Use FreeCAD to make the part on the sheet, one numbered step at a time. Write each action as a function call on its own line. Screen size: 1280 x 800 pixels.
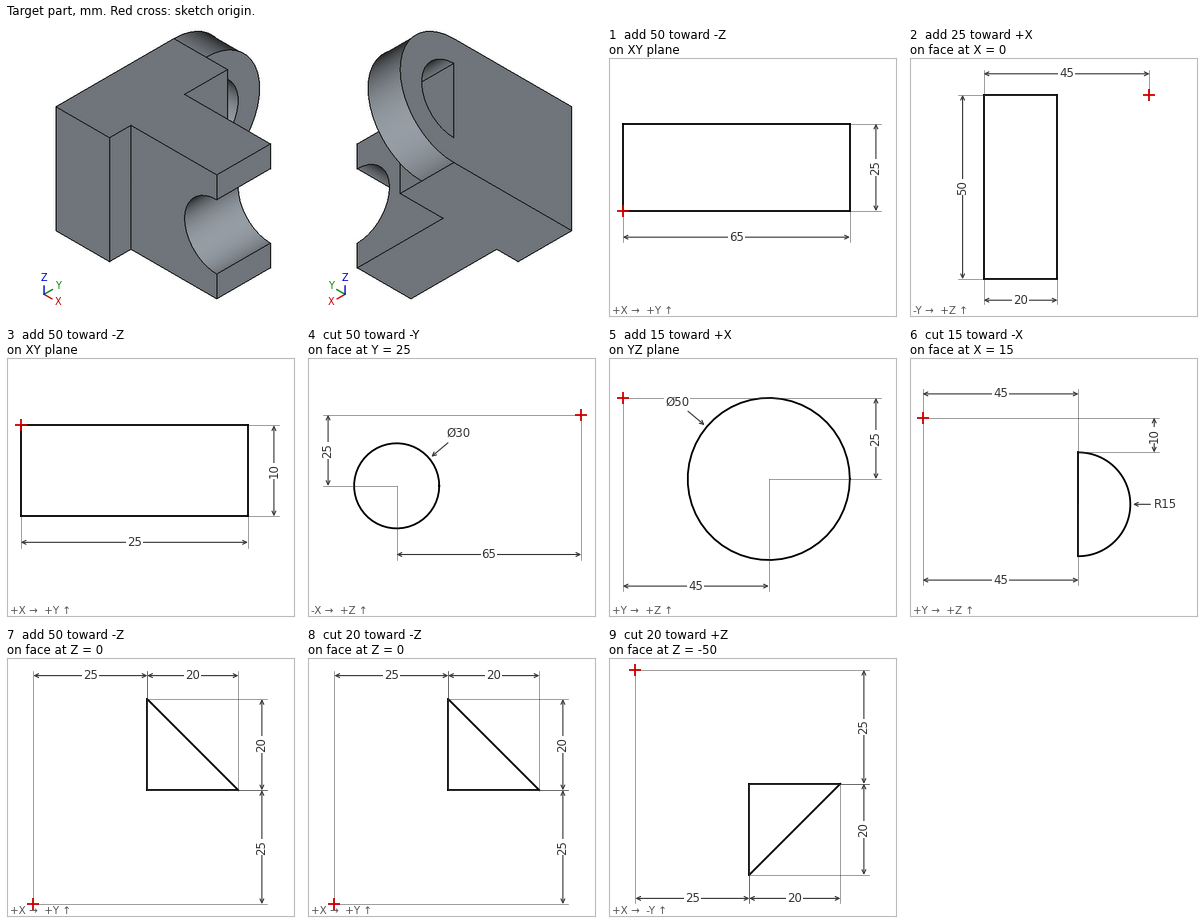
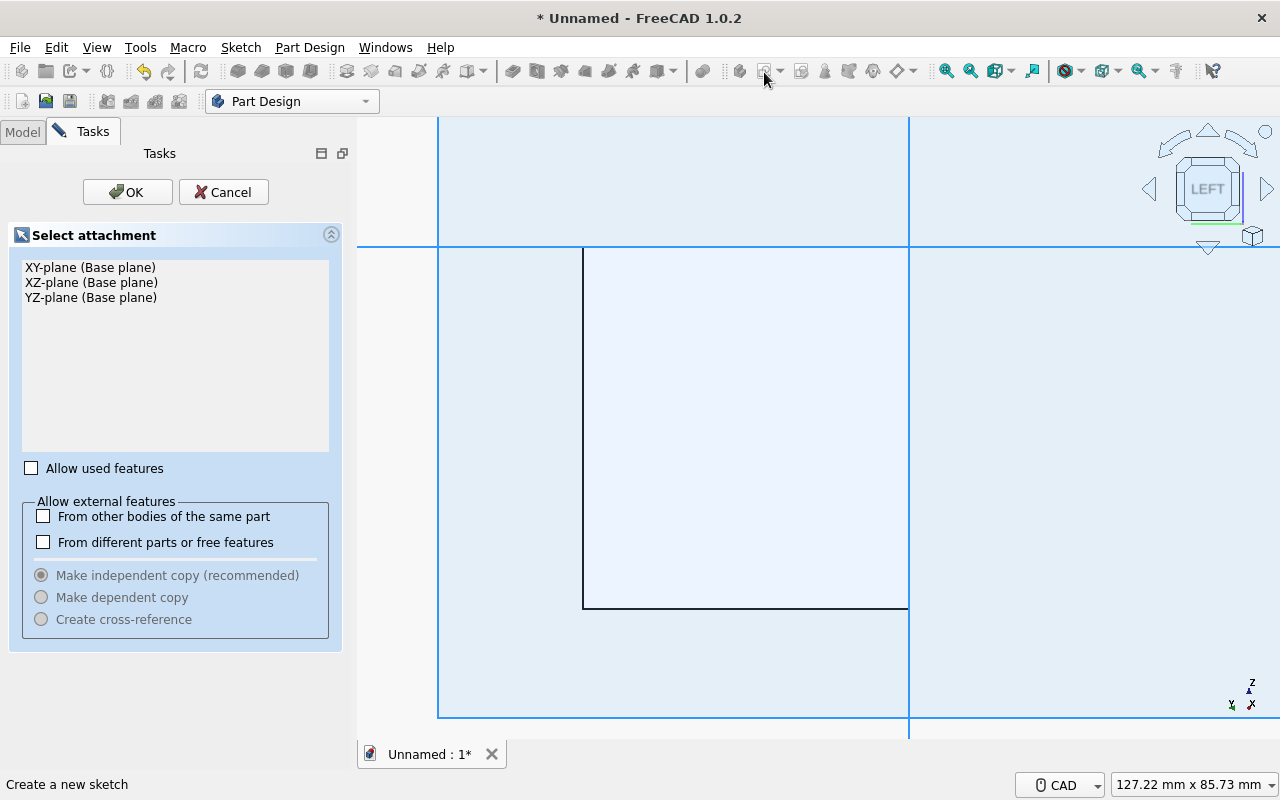
click(82, 268)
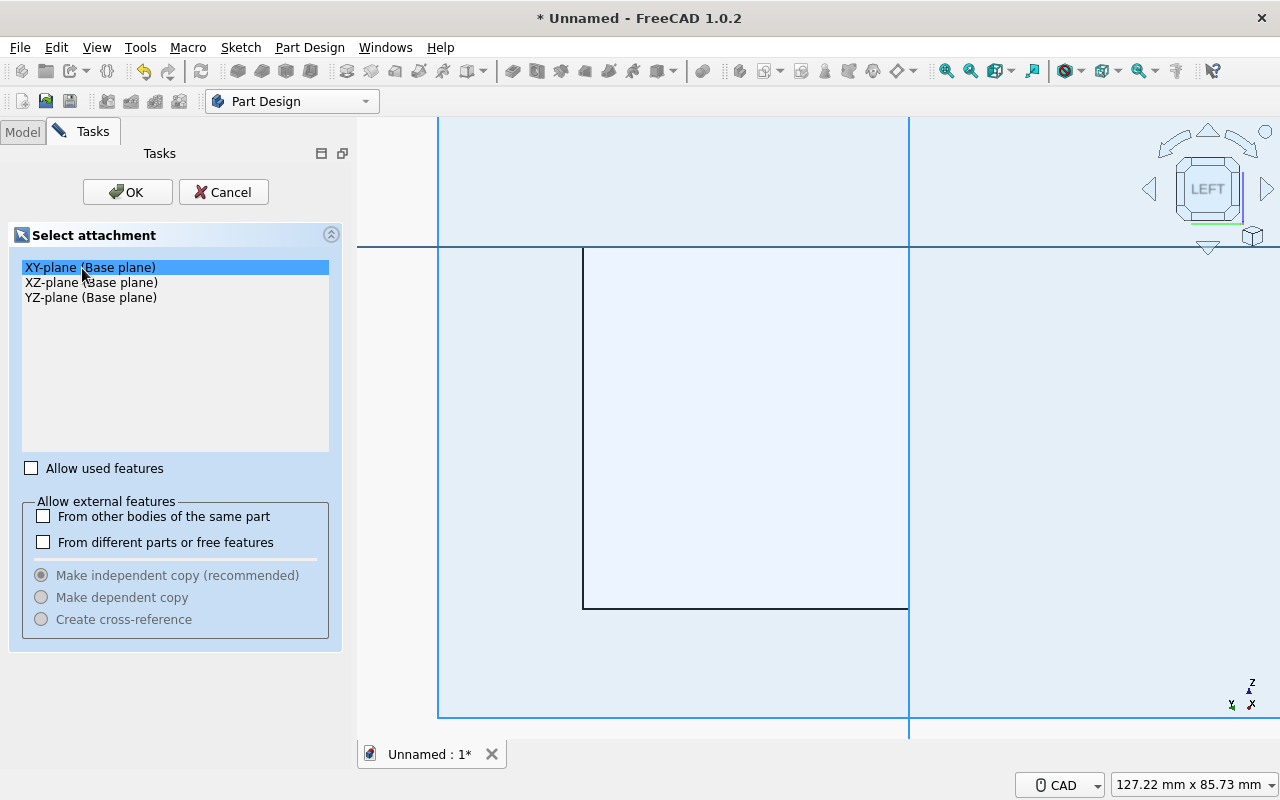
click(128, 192)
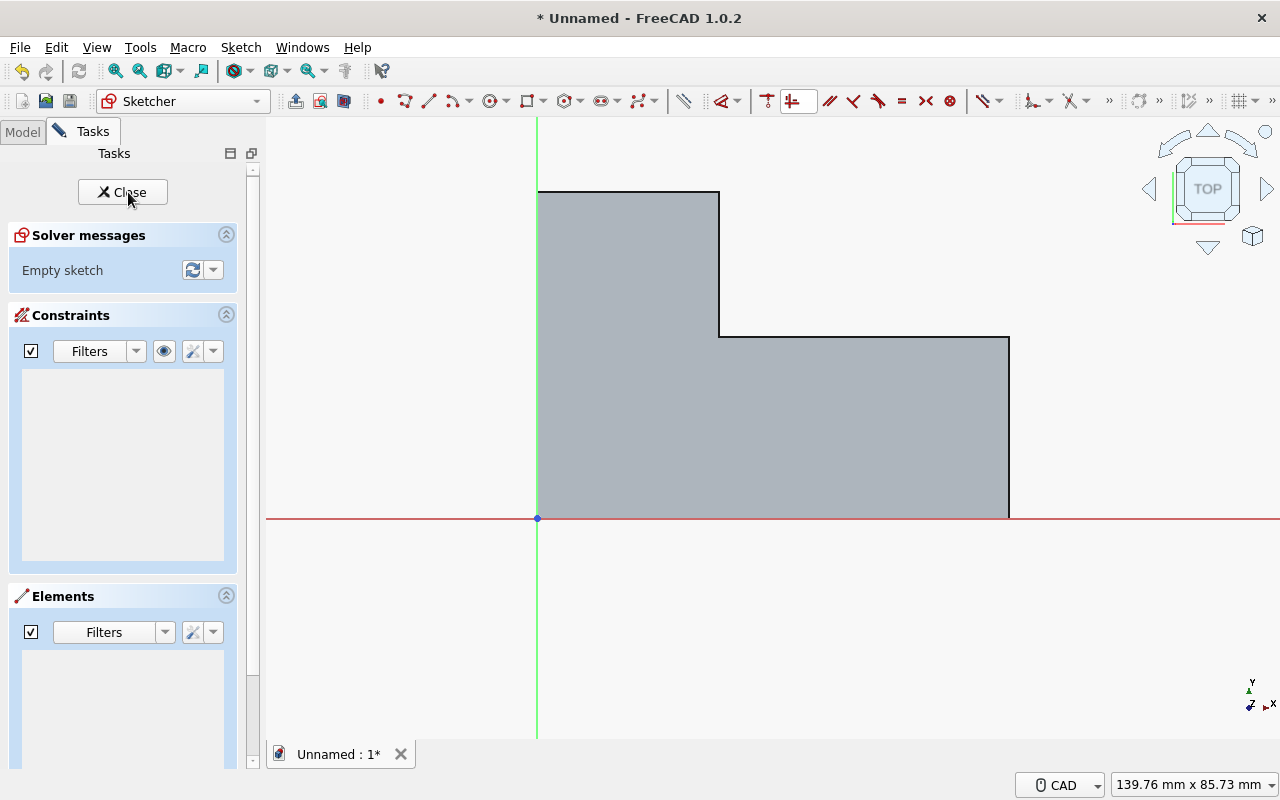
scroll(595, 610, up, 6)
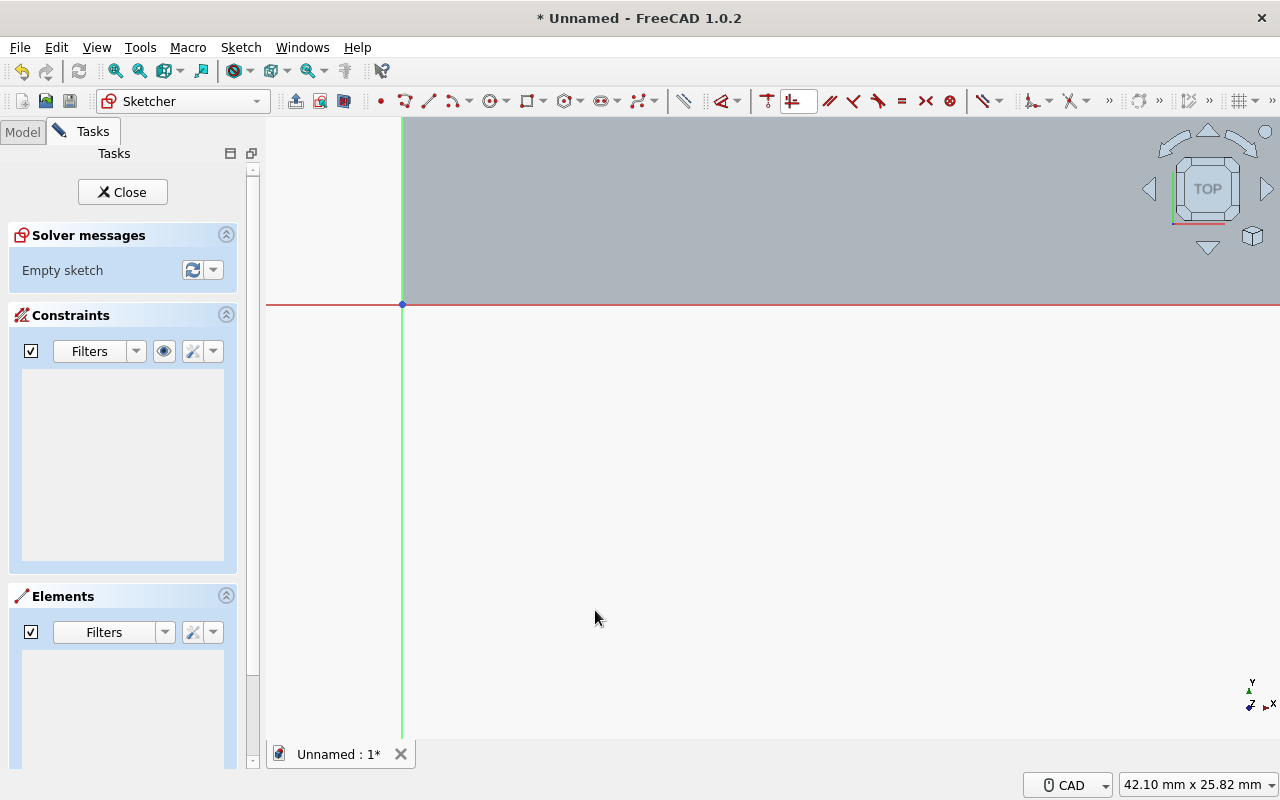
click(528, 102)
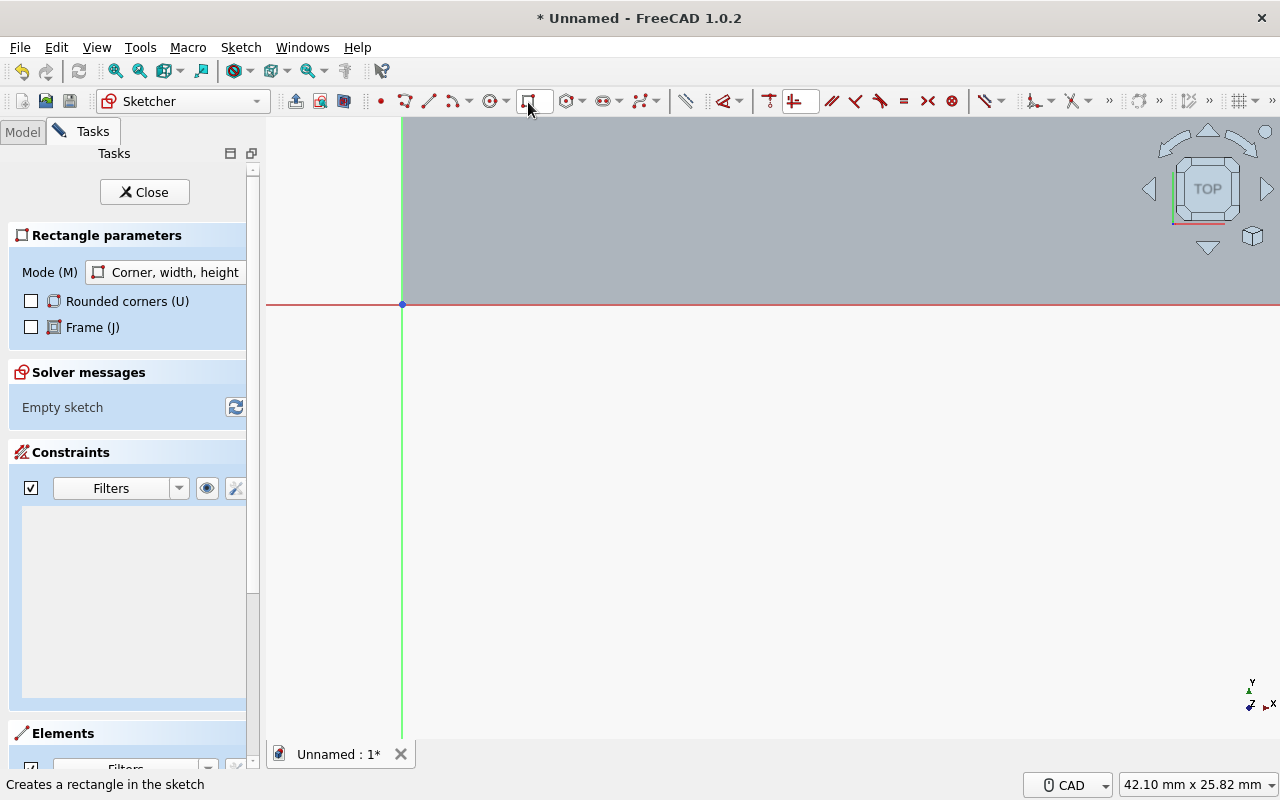
click(402, 305)
move(1005, 546)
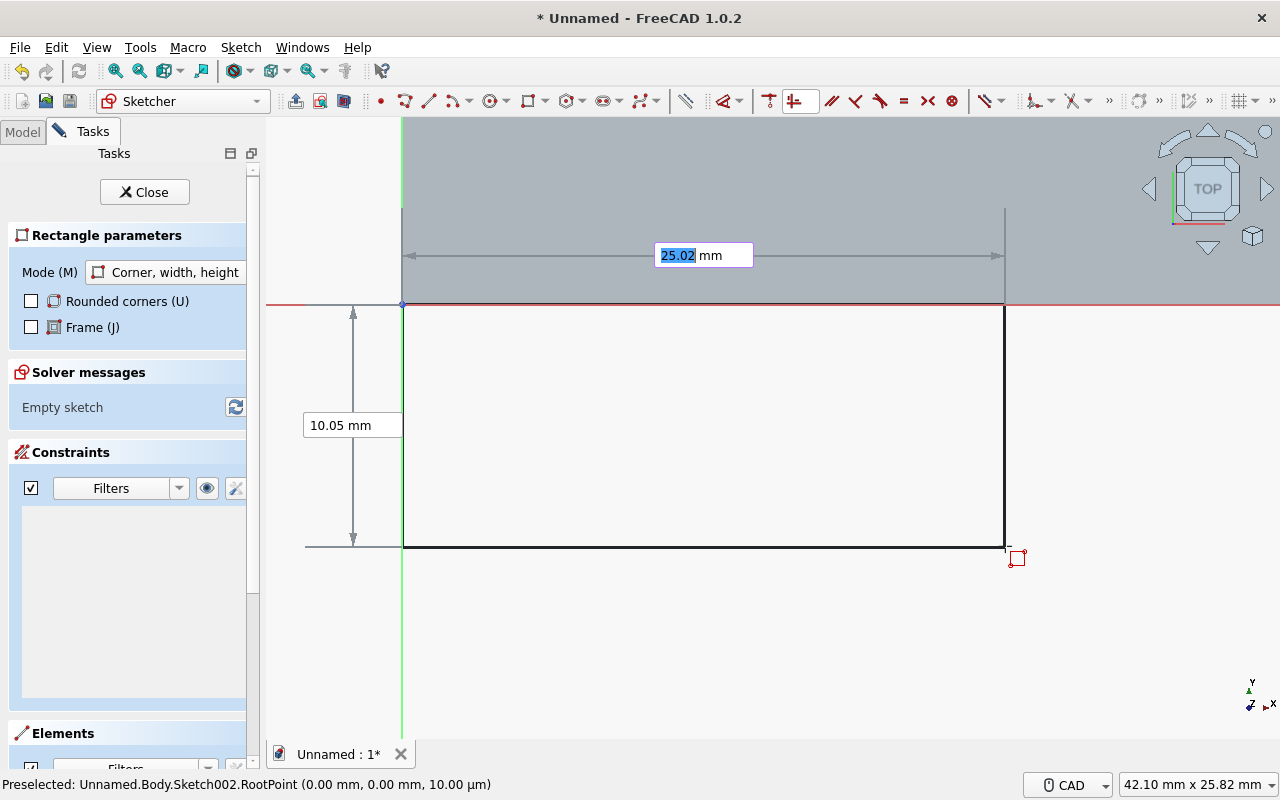
text(25)
key(Tab)
text(10)
key(Return)
key(Escape)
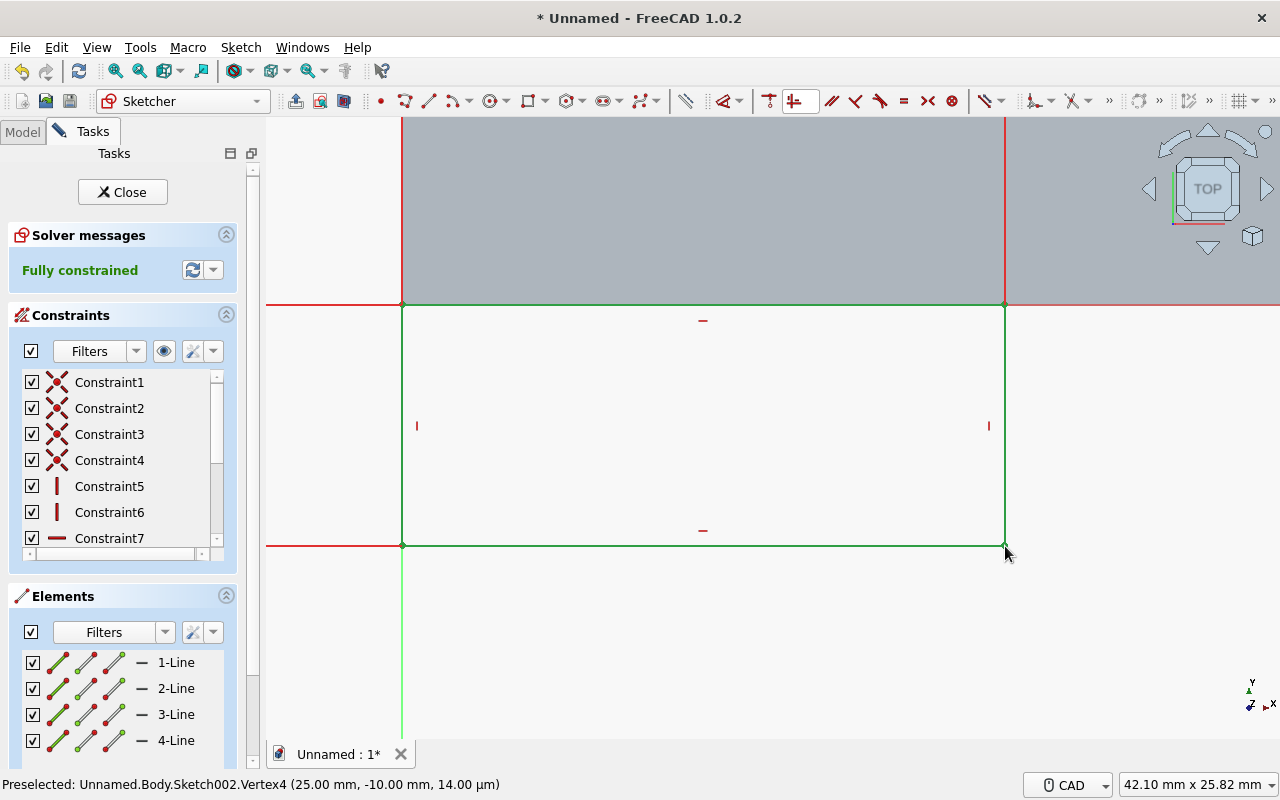
click(123, 192)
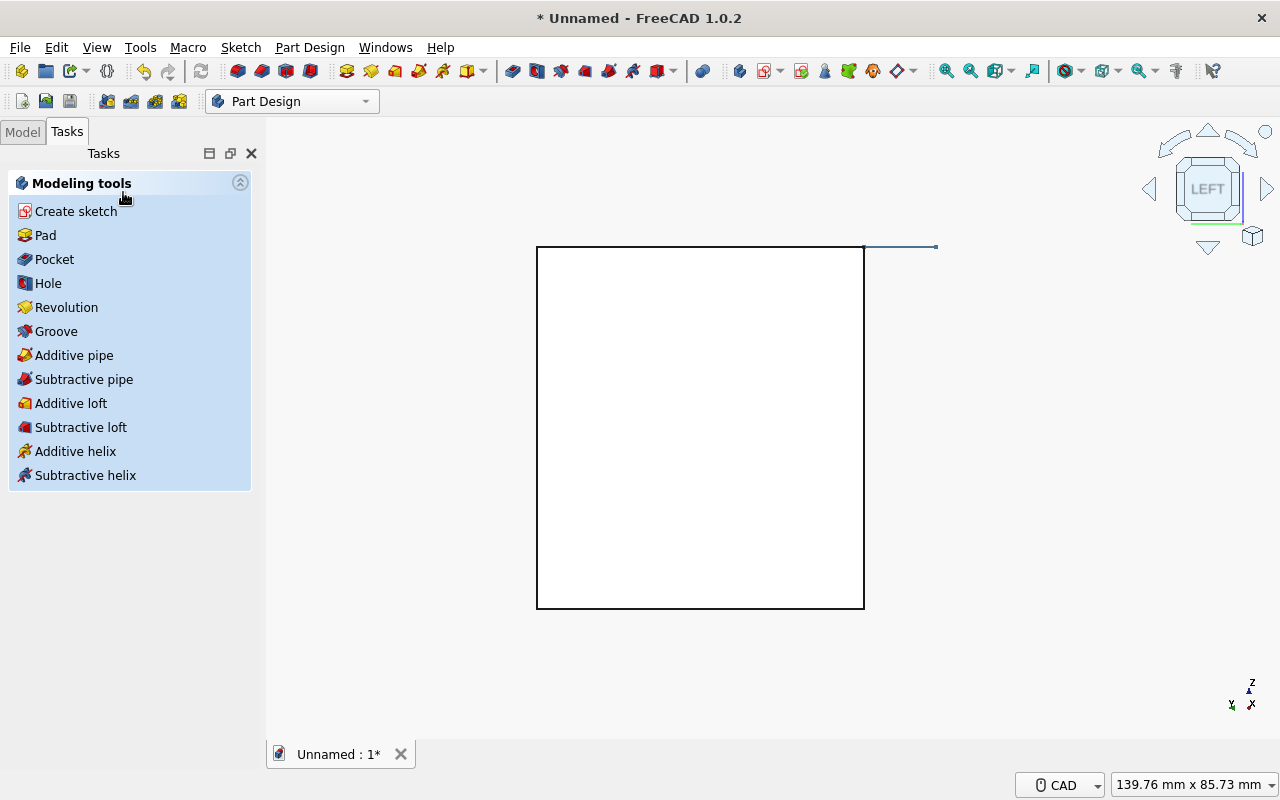
click(348, 72)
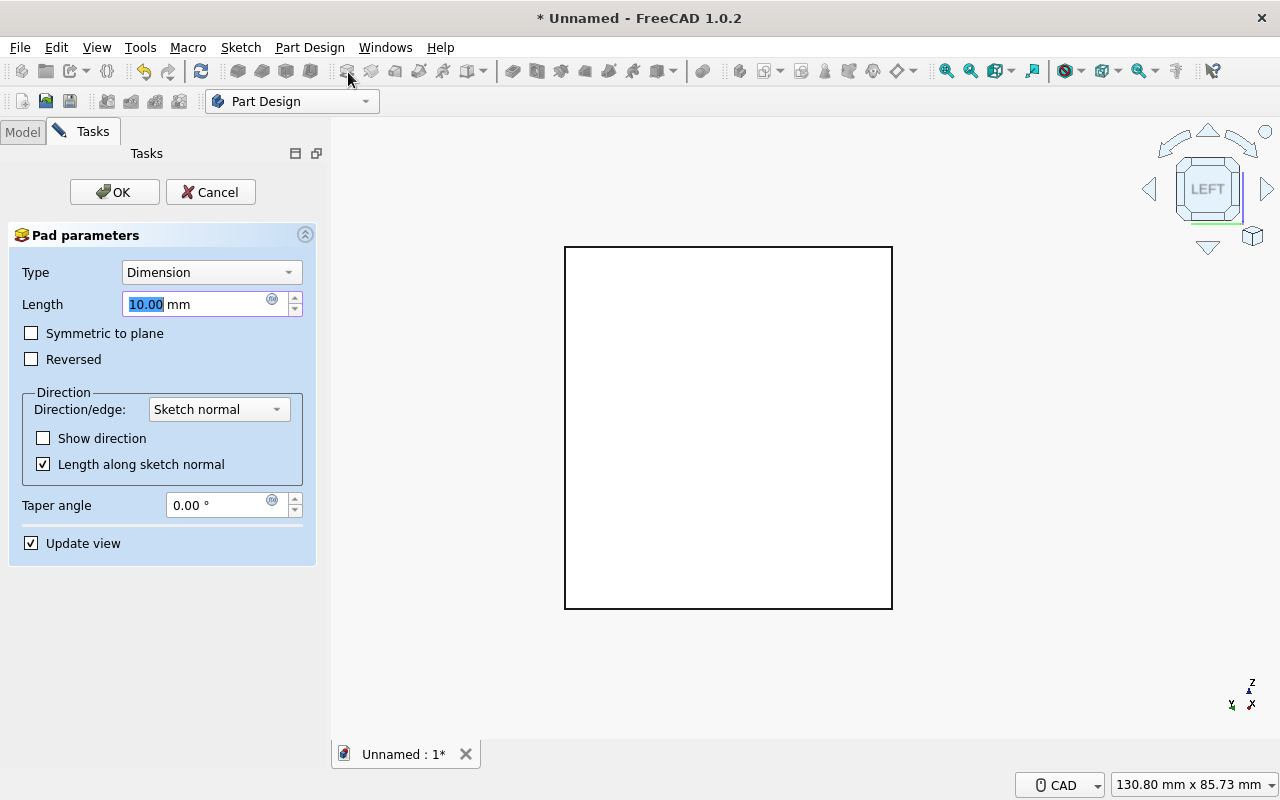
text(50)
key(Tab)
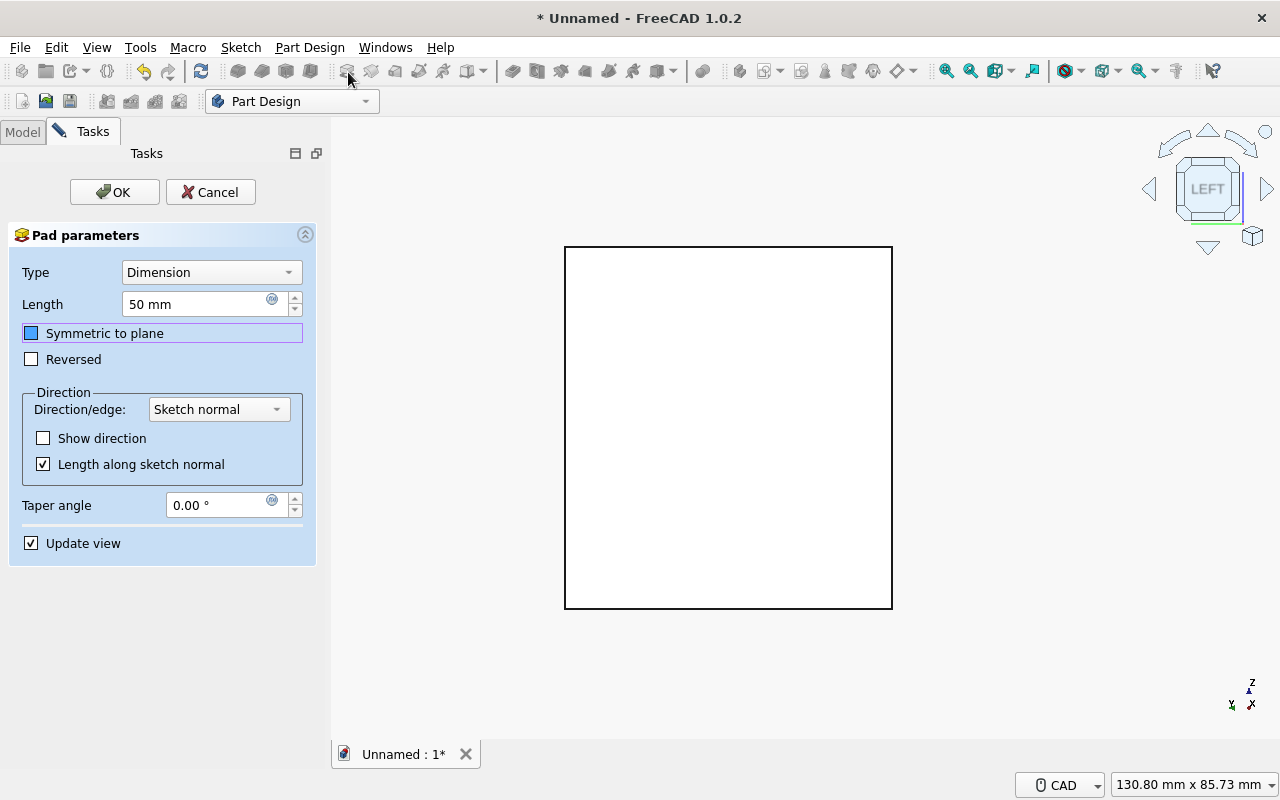
click(30, 359)